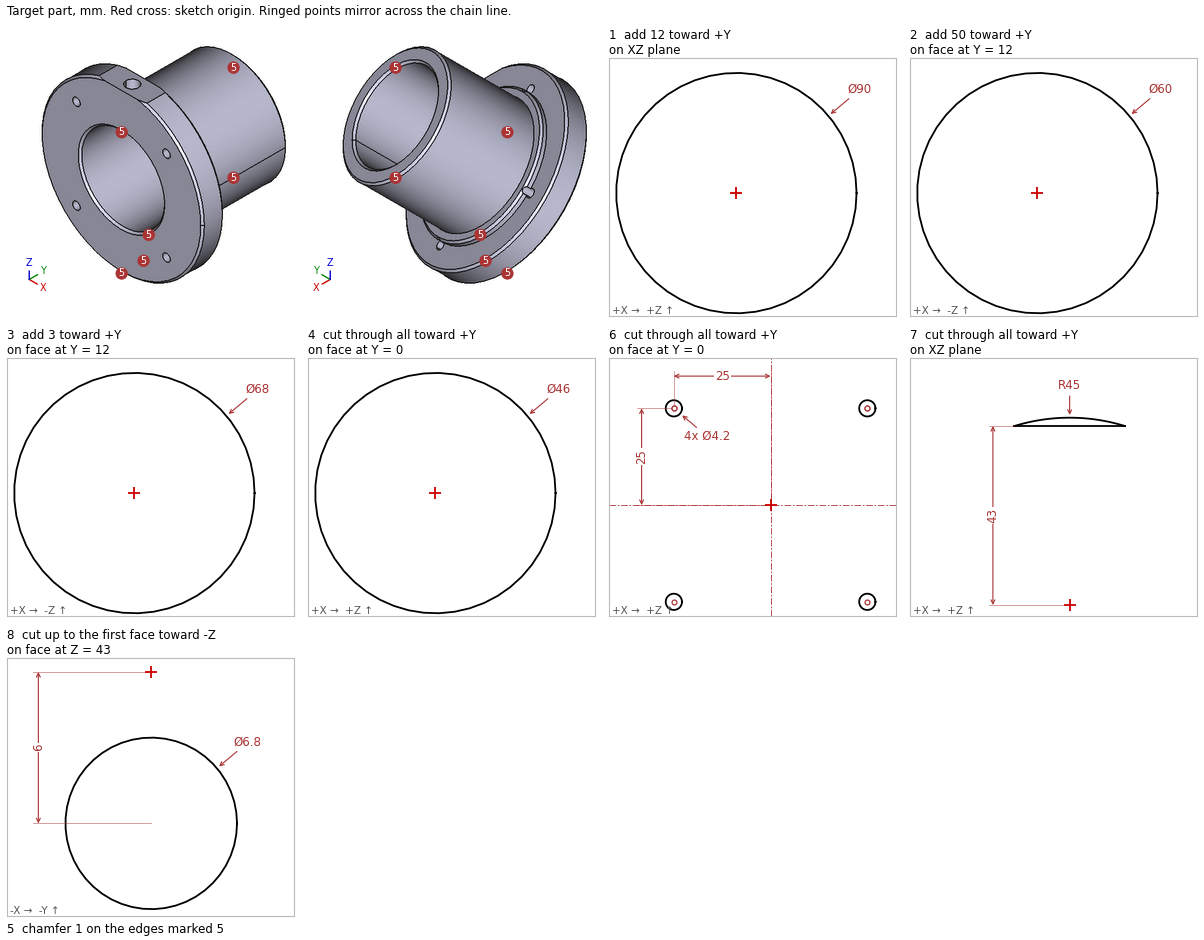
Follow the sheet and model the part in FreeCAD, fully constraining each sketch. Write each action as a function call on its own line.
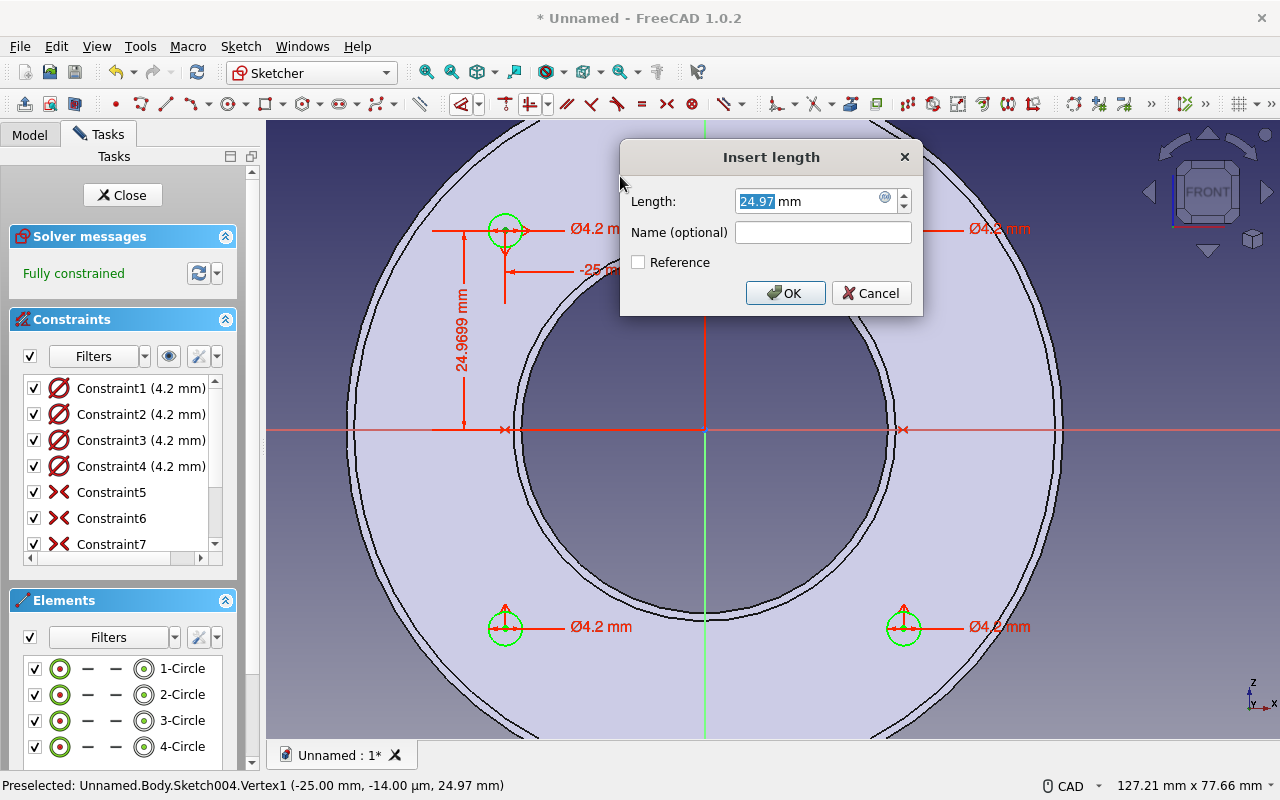
text(25)
key(Return)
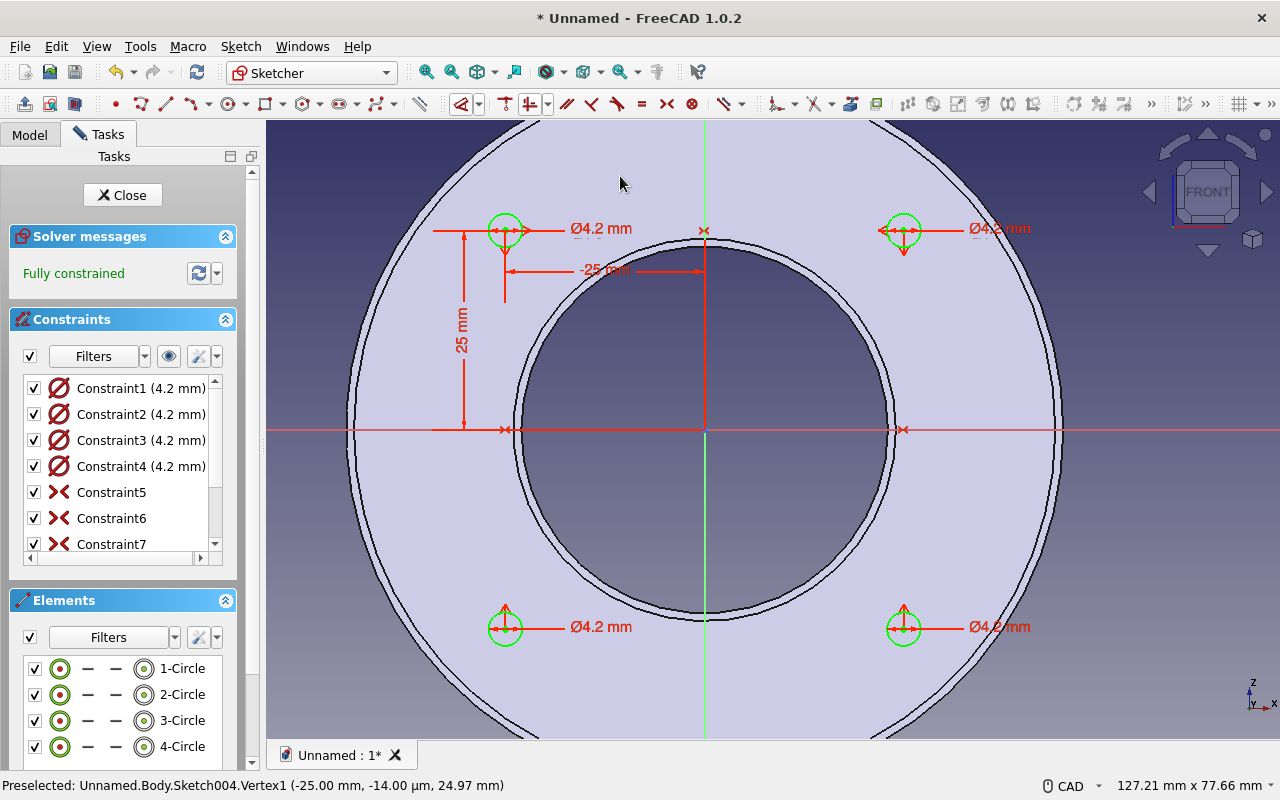
click(123, 195)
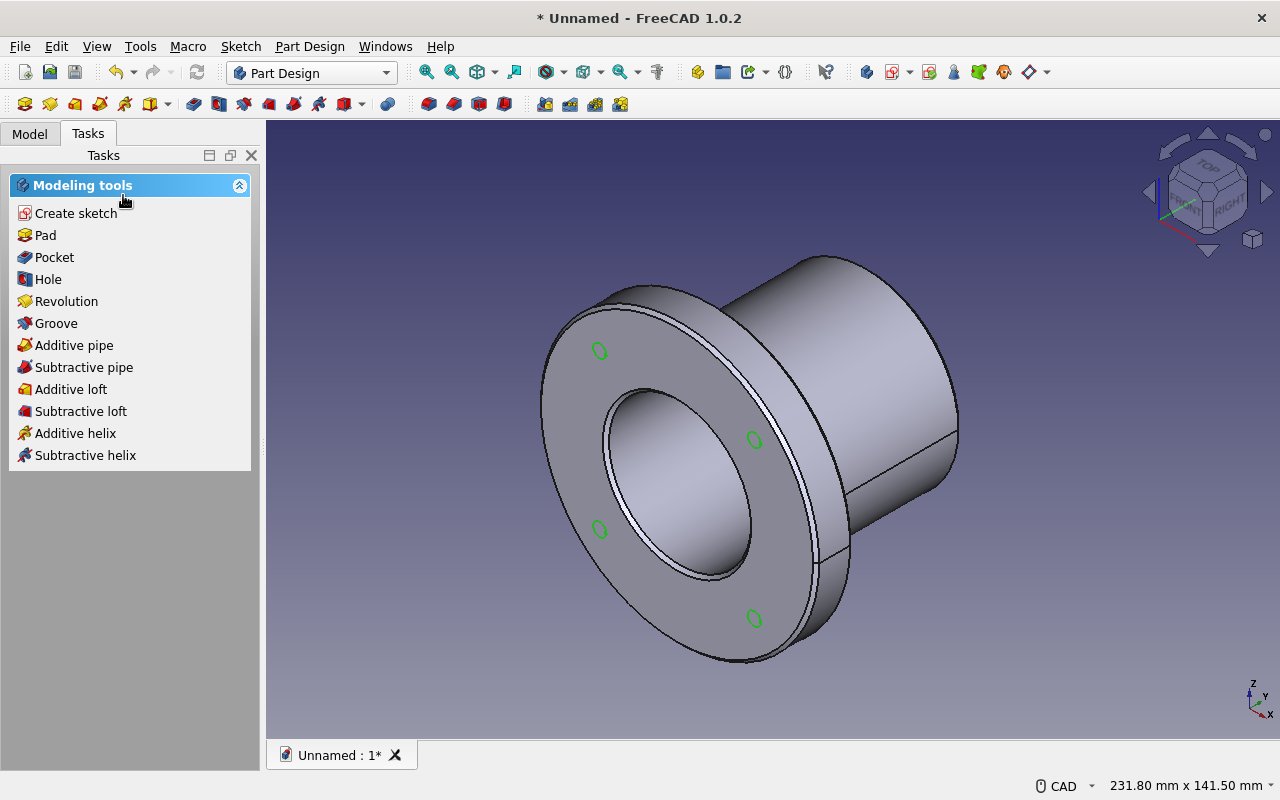
click(194, 104)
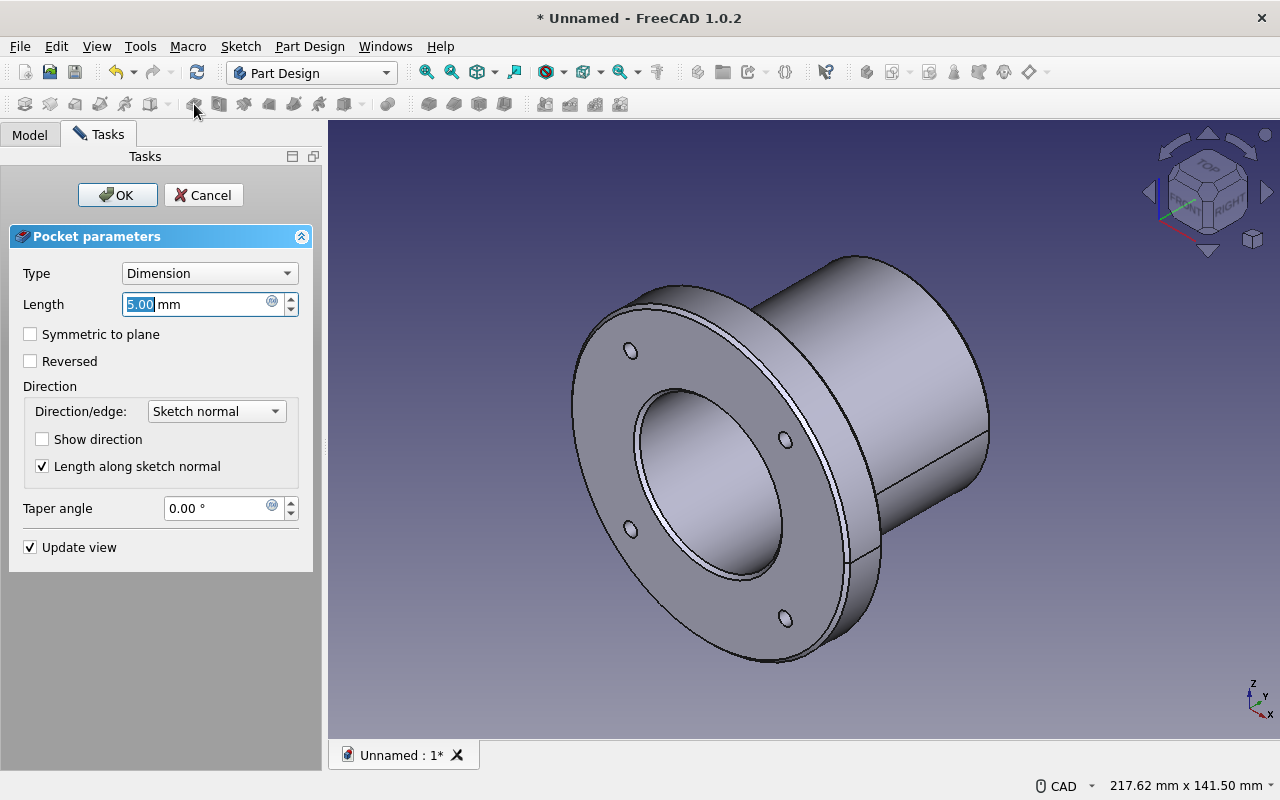
click(210, 274)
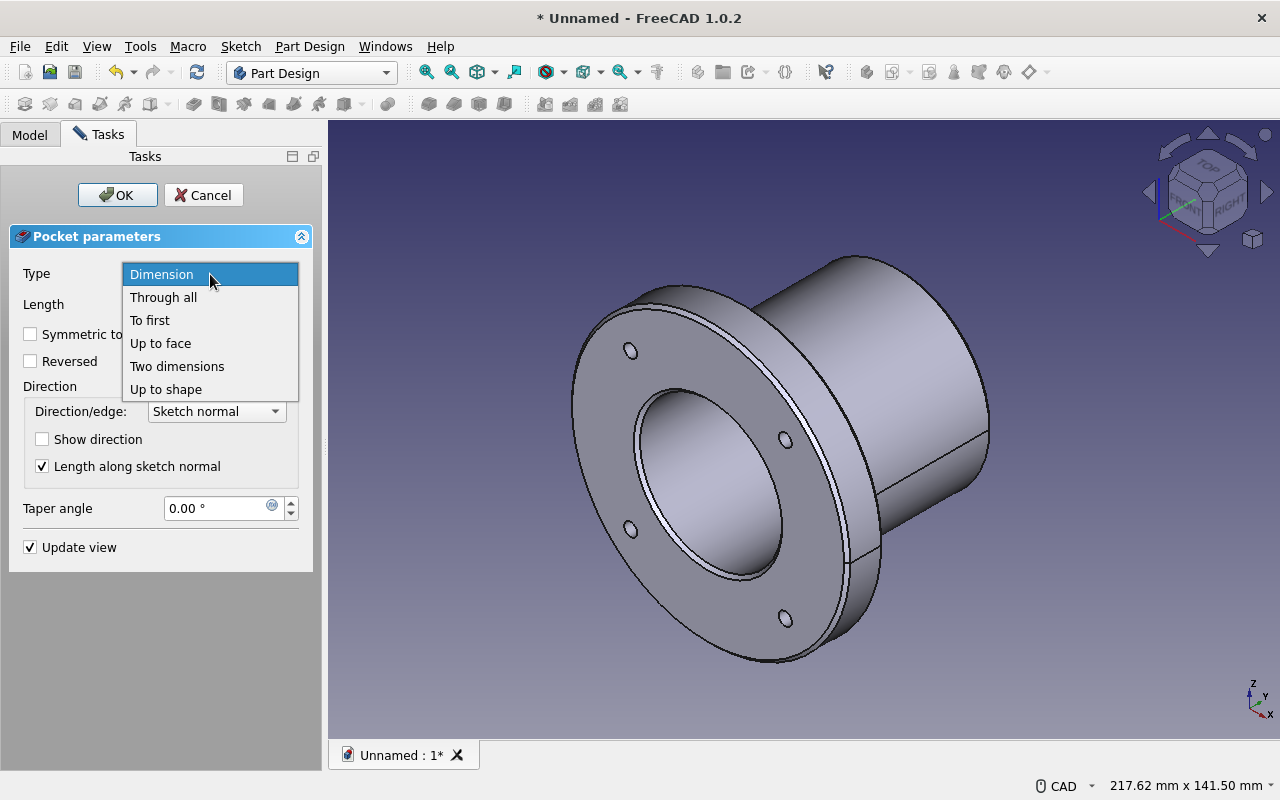
click(208, 298)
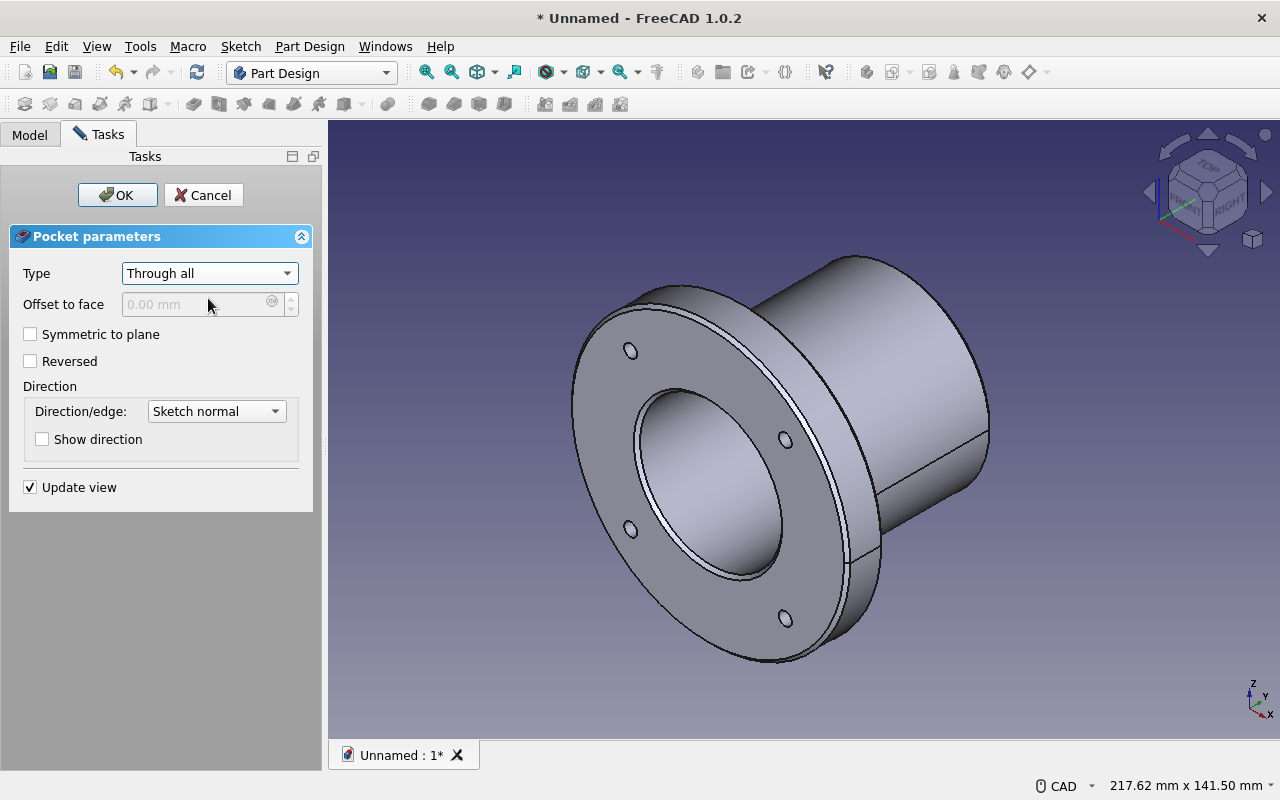
click(118, 195)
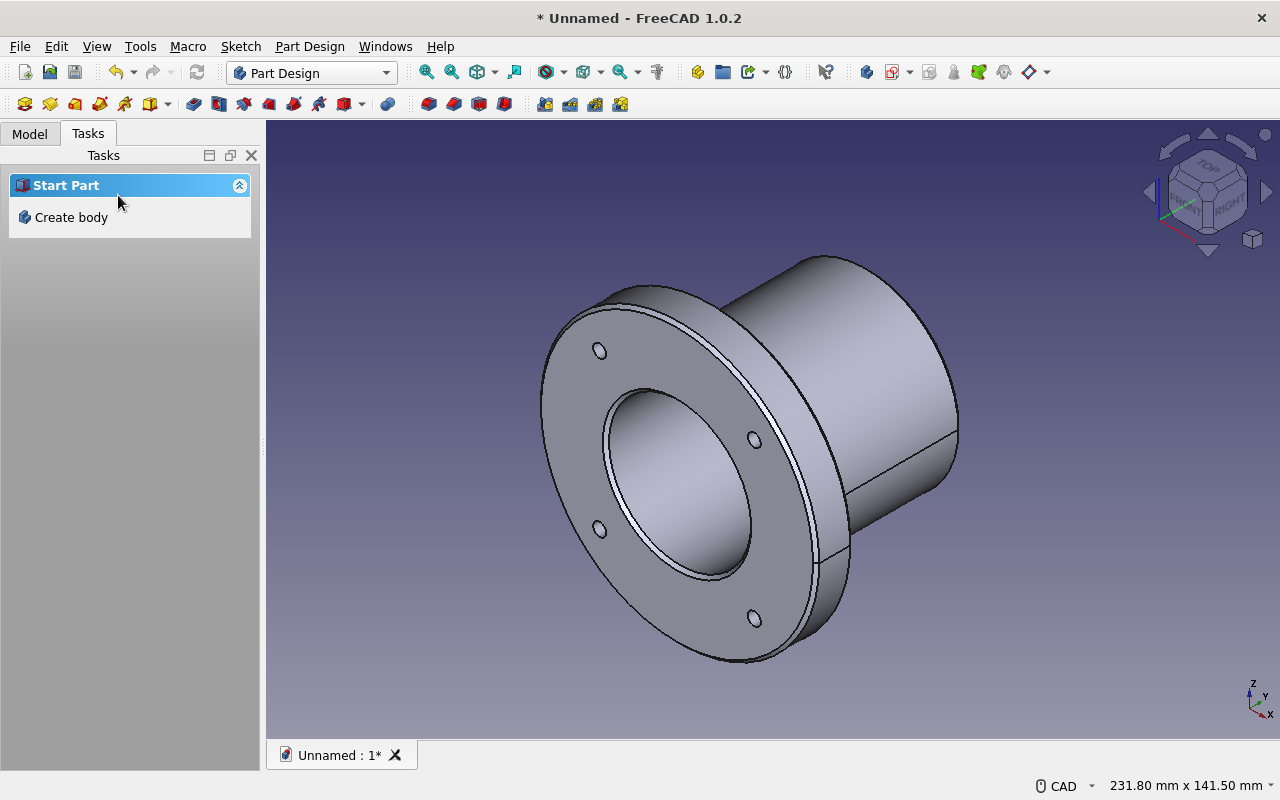
click(892, 72)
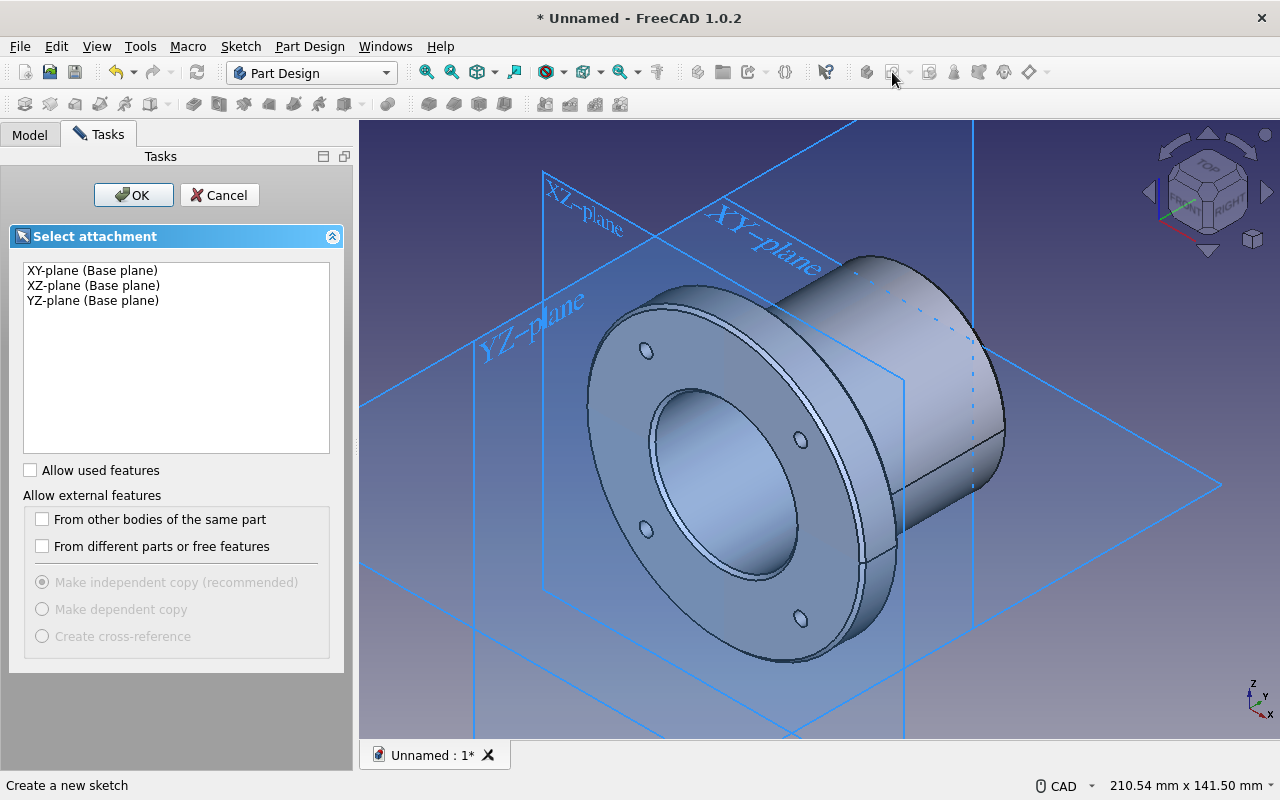
click(84, 286)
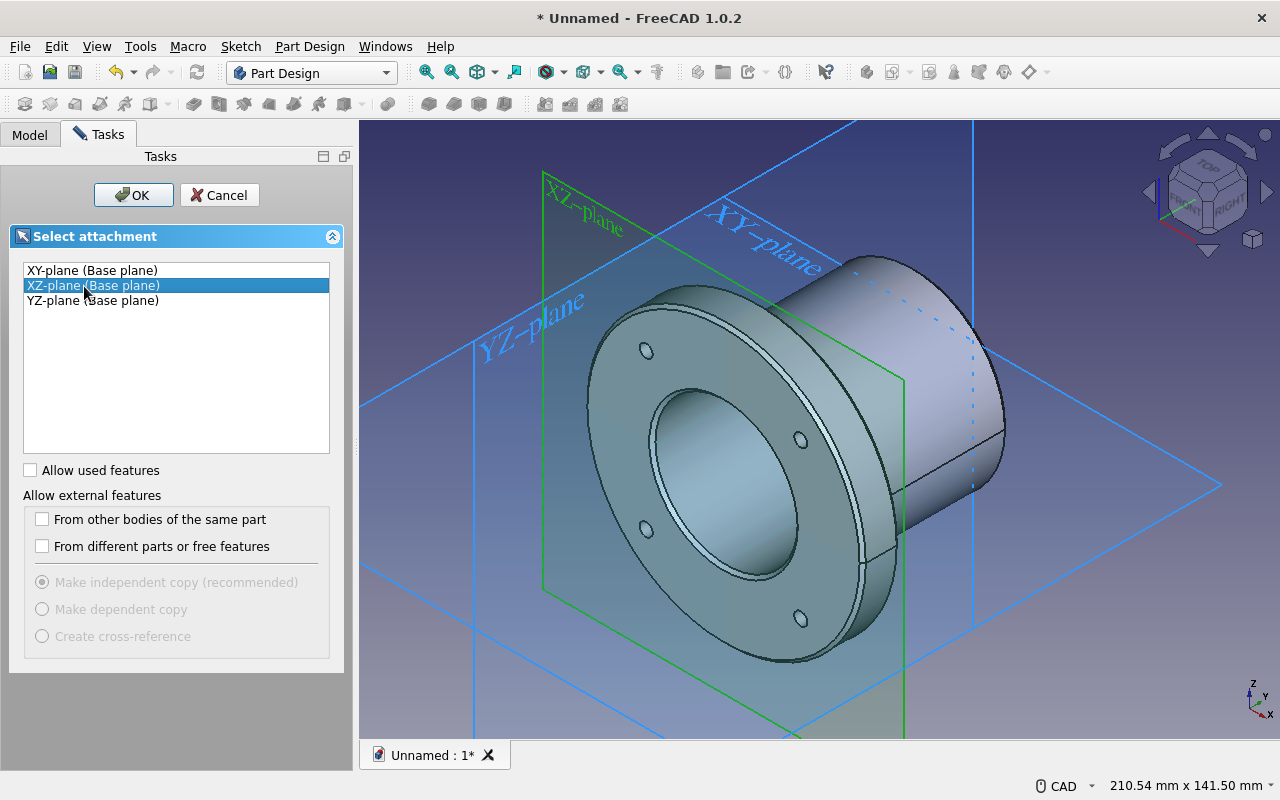
click(134, 195)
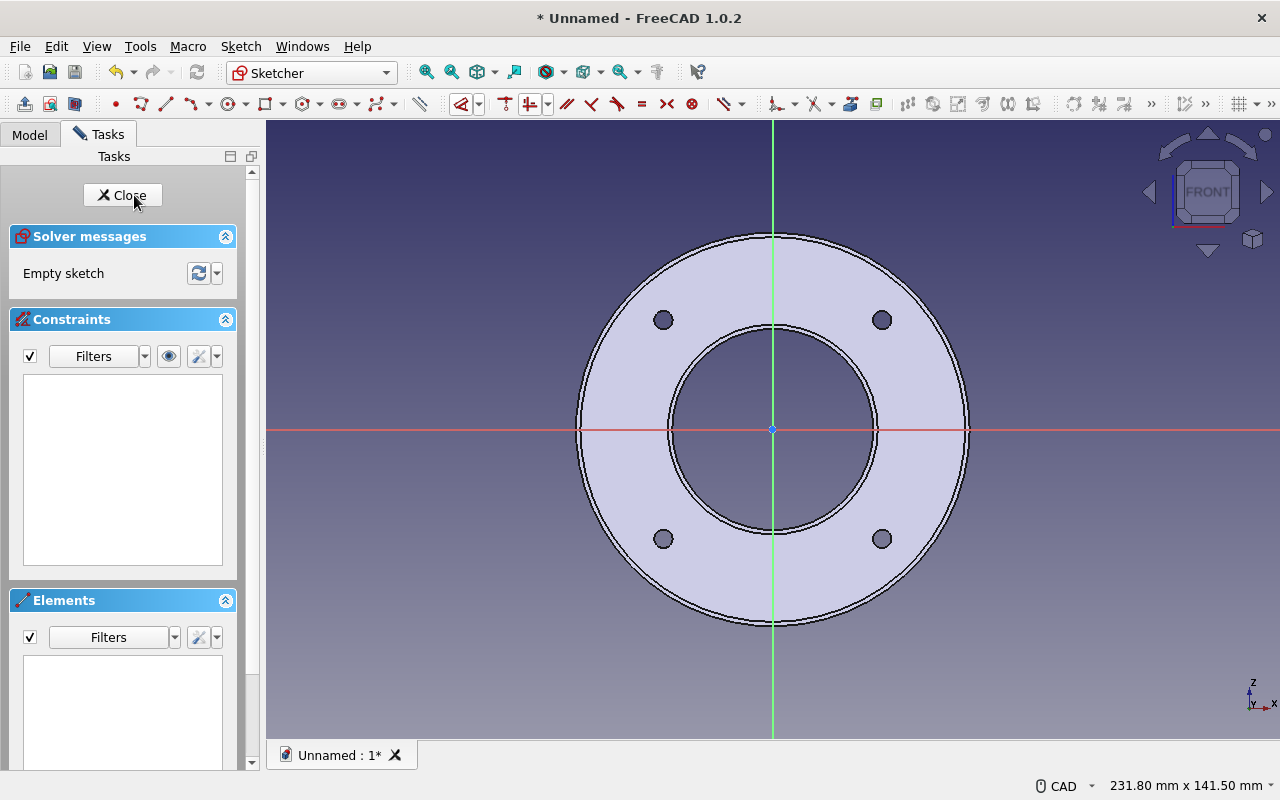
scroll(829, 251, up, 4)